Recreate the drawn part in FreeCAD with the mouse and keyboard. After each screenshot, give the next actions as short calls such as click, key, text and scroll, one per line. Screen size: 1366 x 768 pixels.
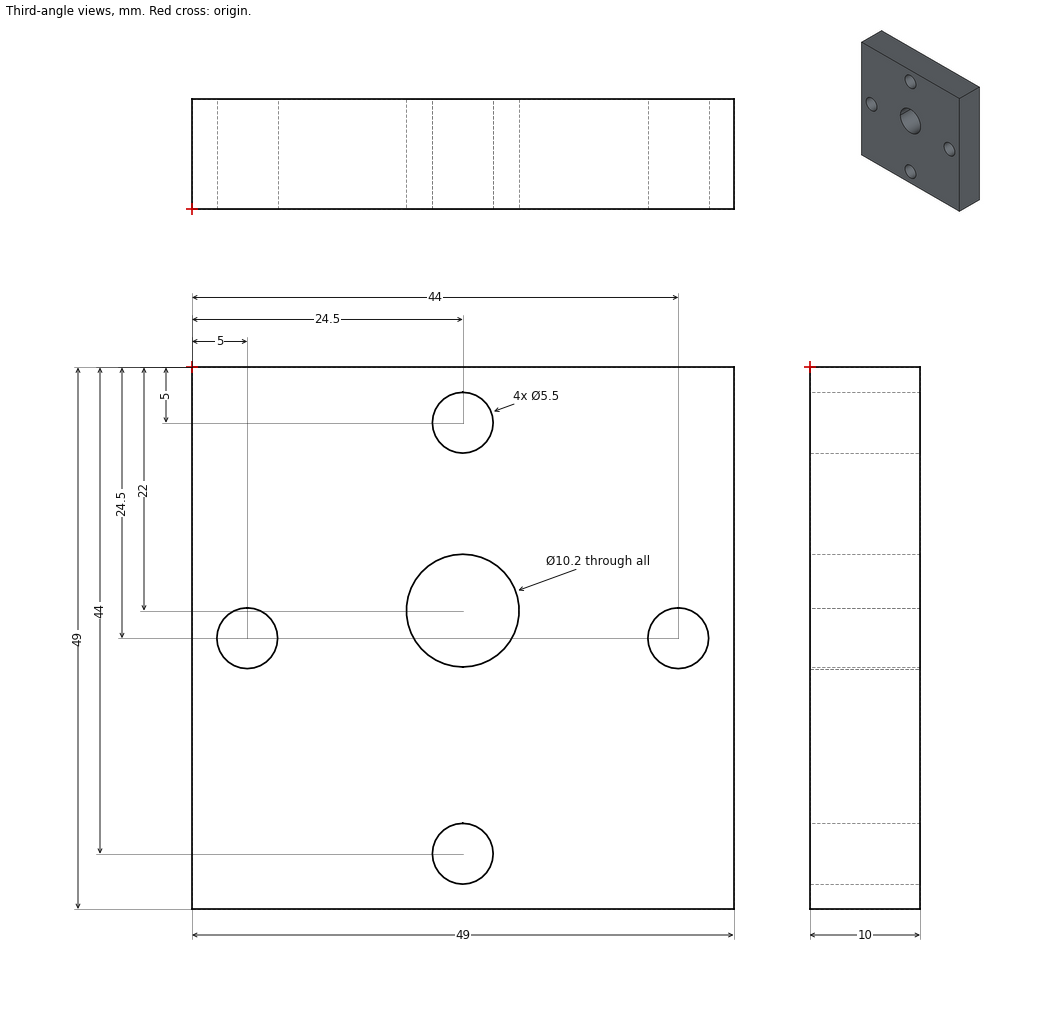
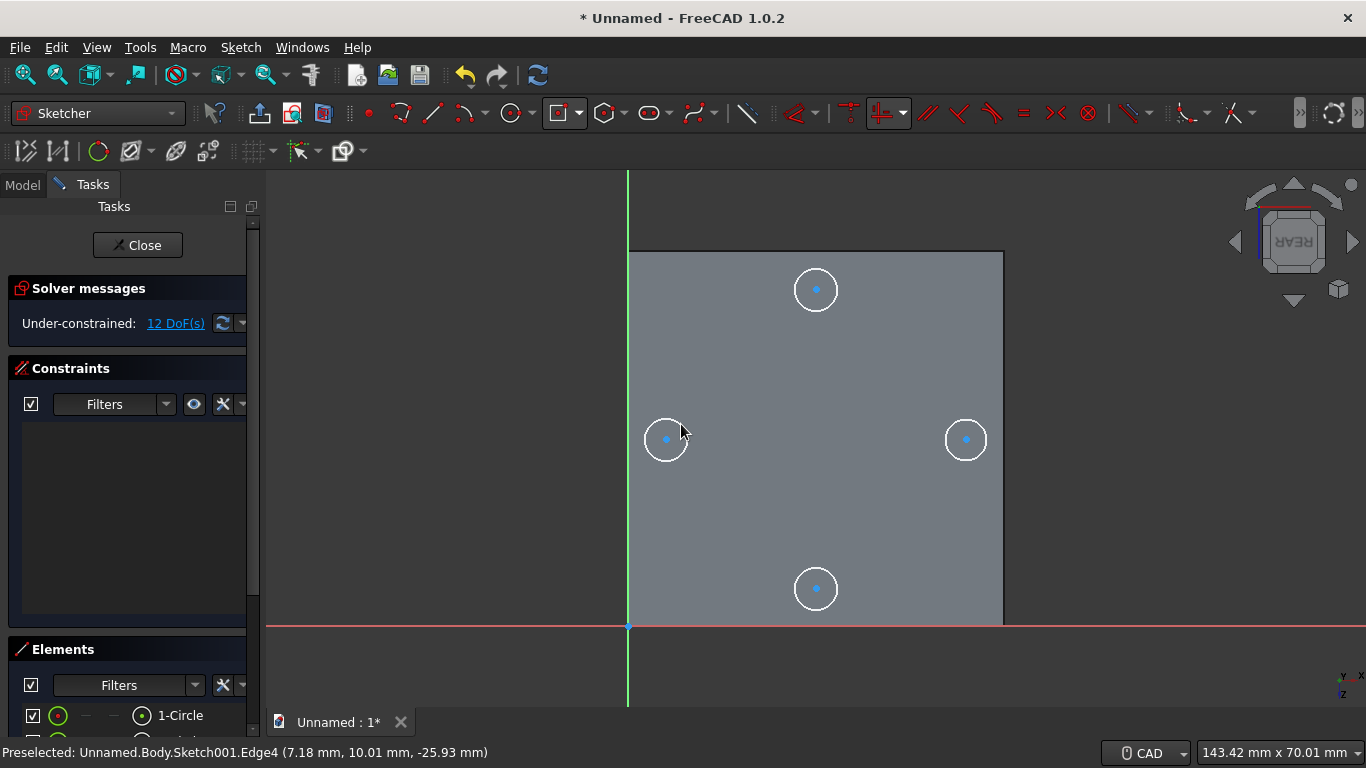
click(831, 574)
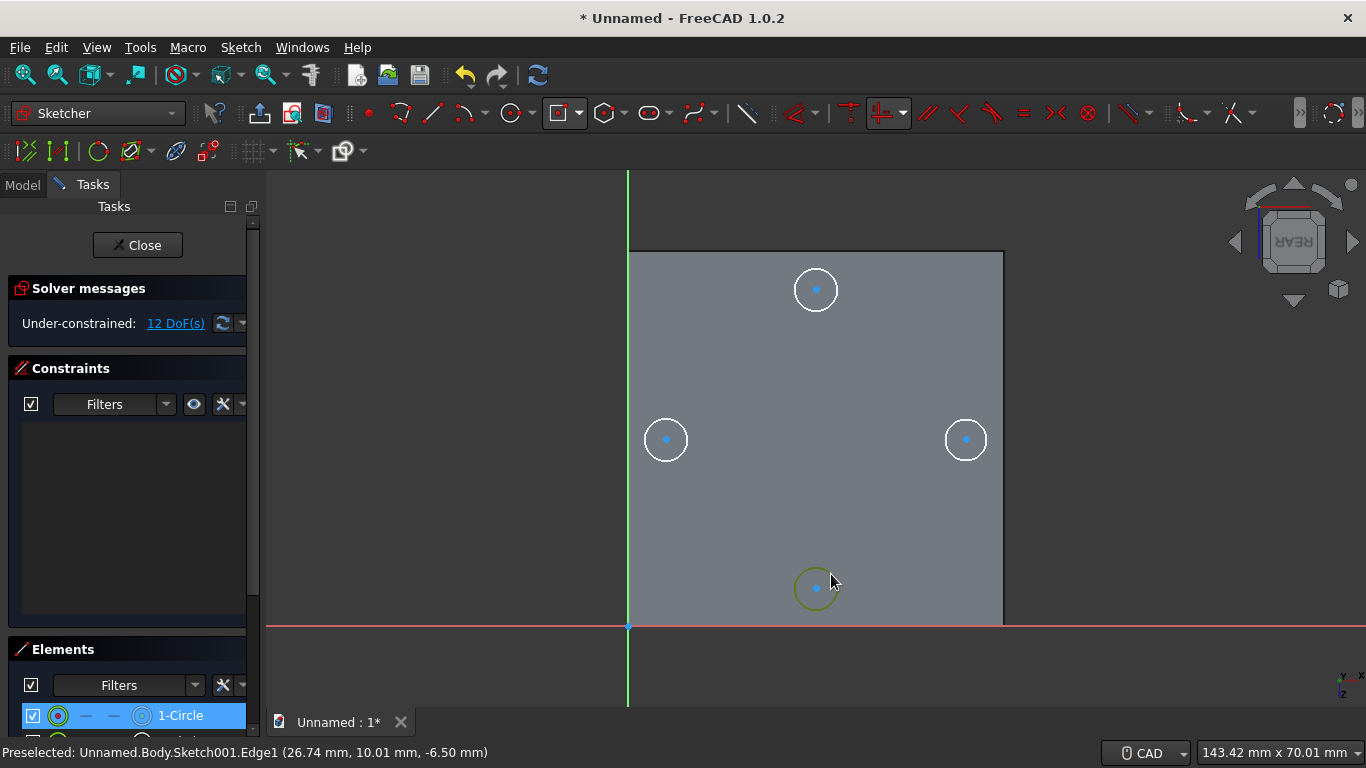
click(980, 425)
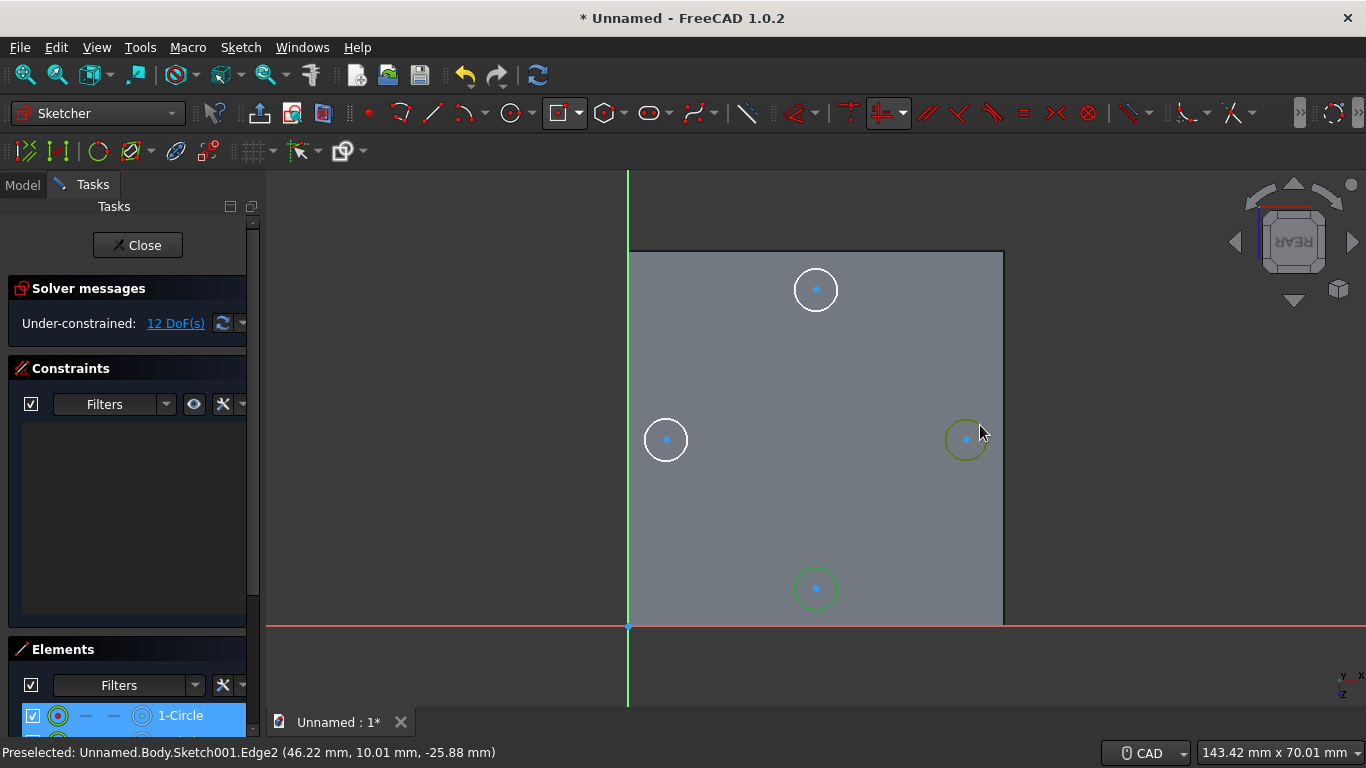
click(831, 275)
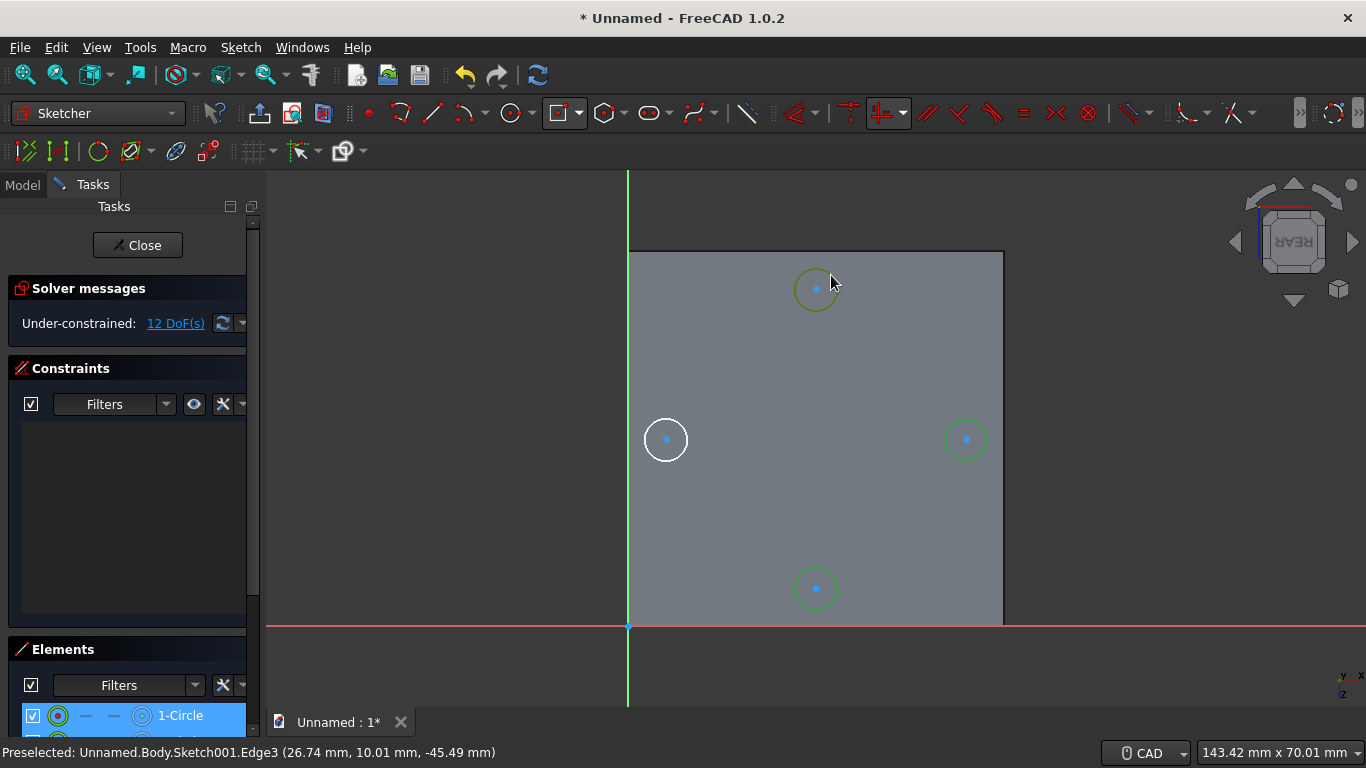
click(681, 425)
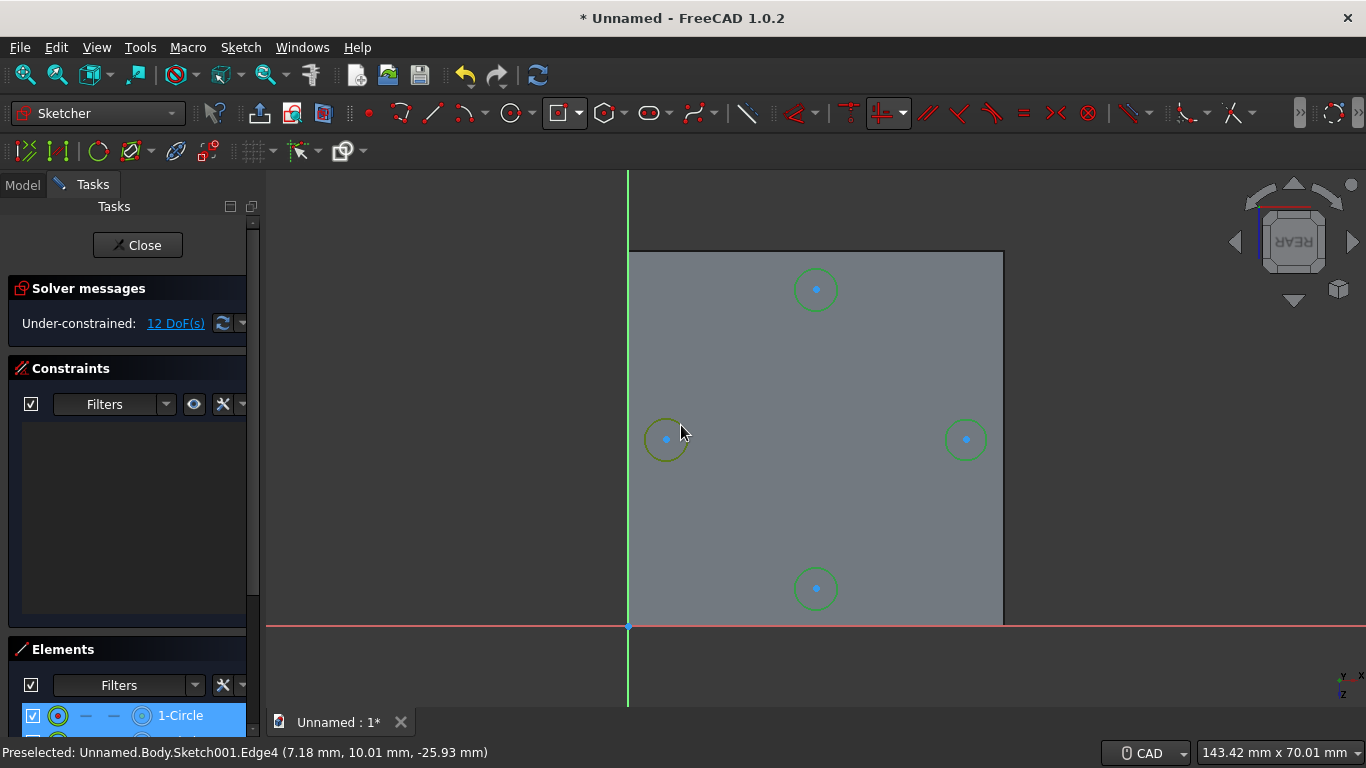
click(1024, 114)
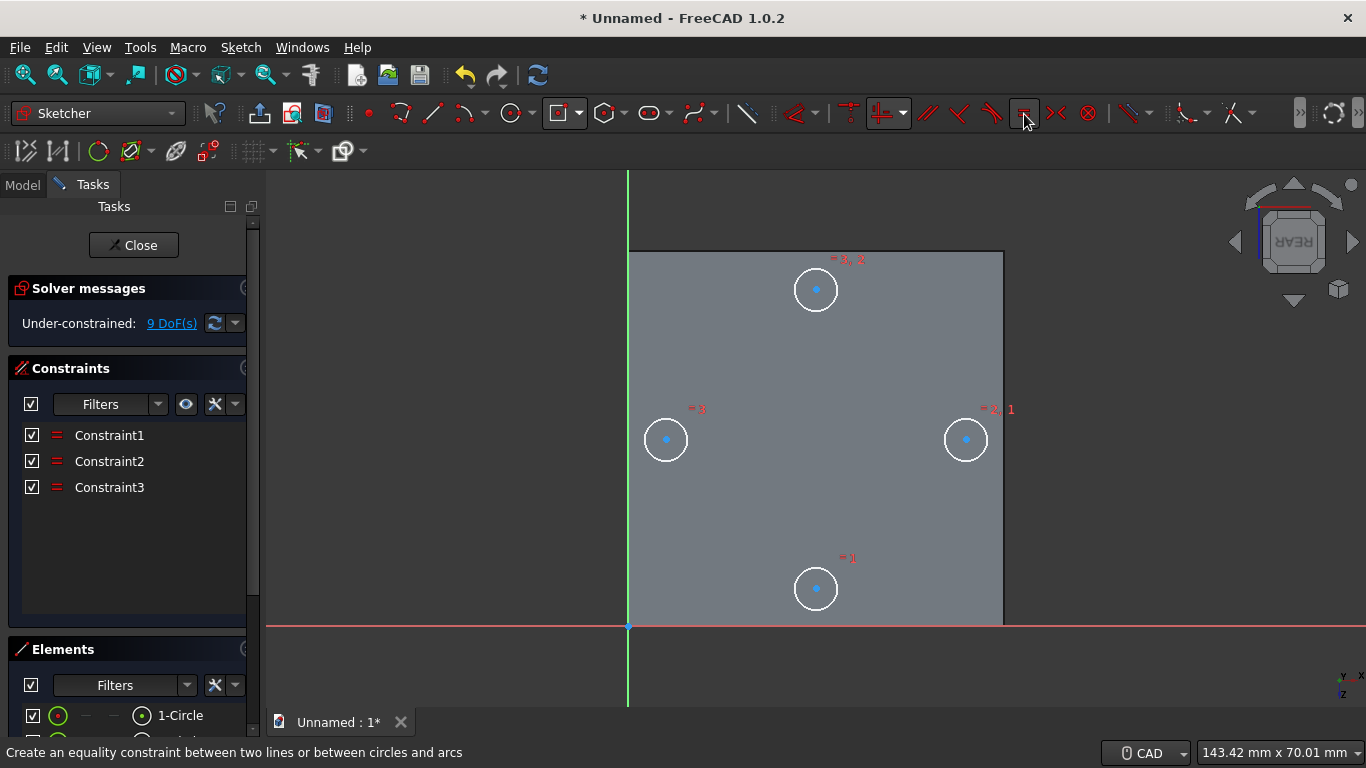
click(816, 589)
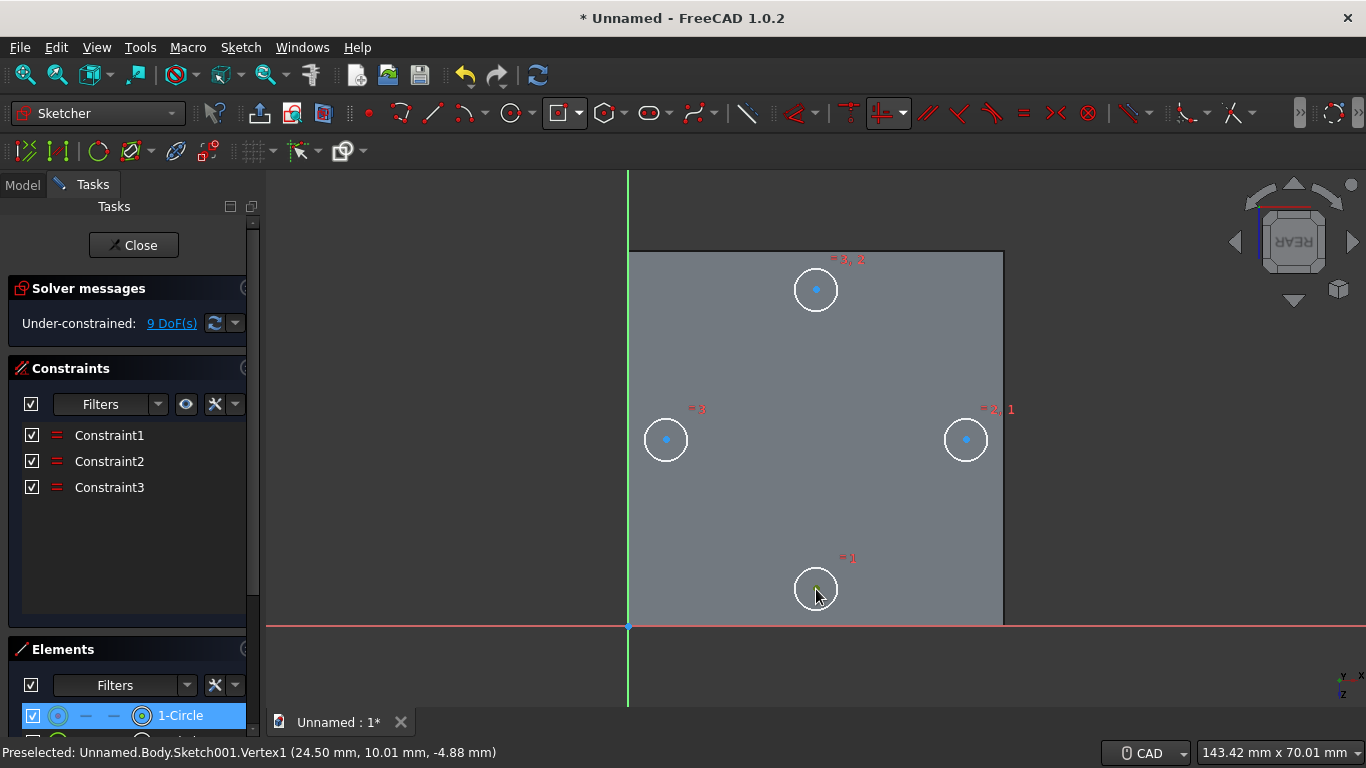
click(816, 290)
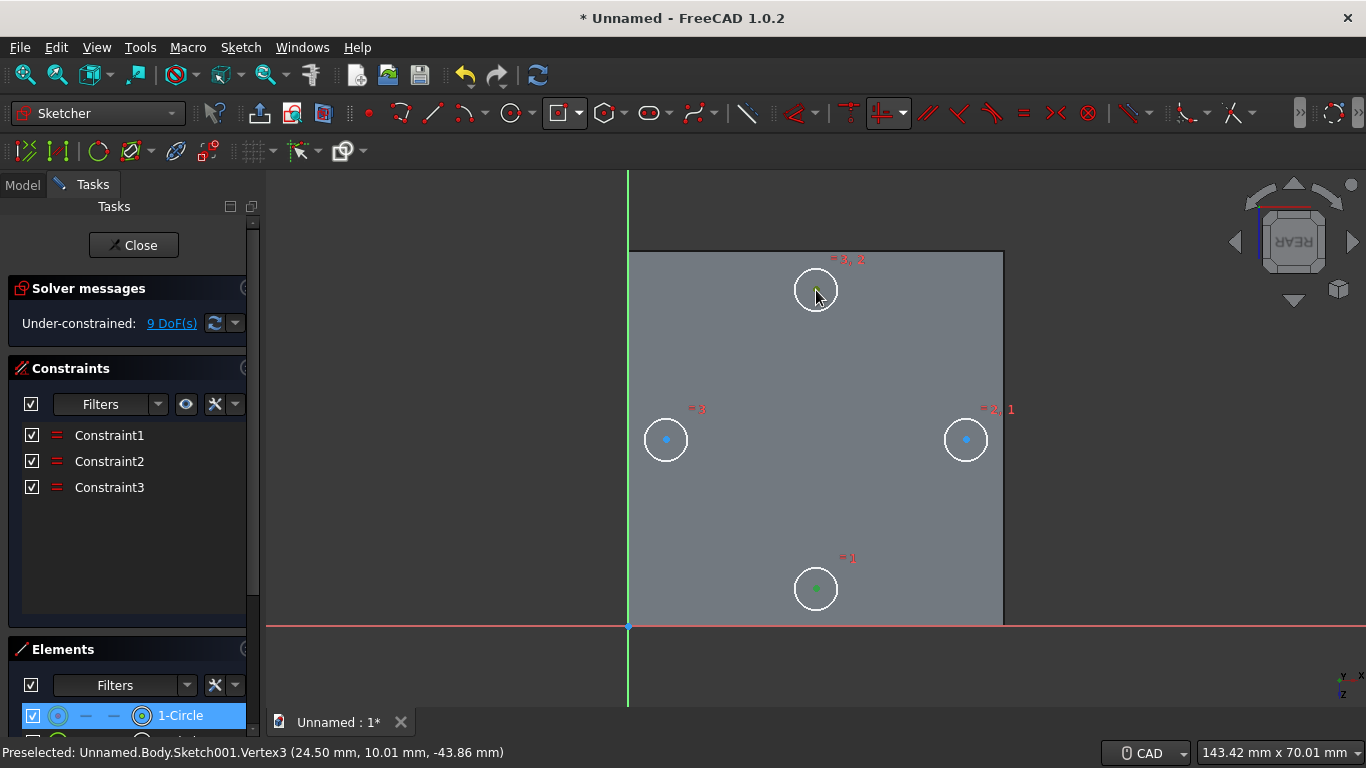
click(906, 114)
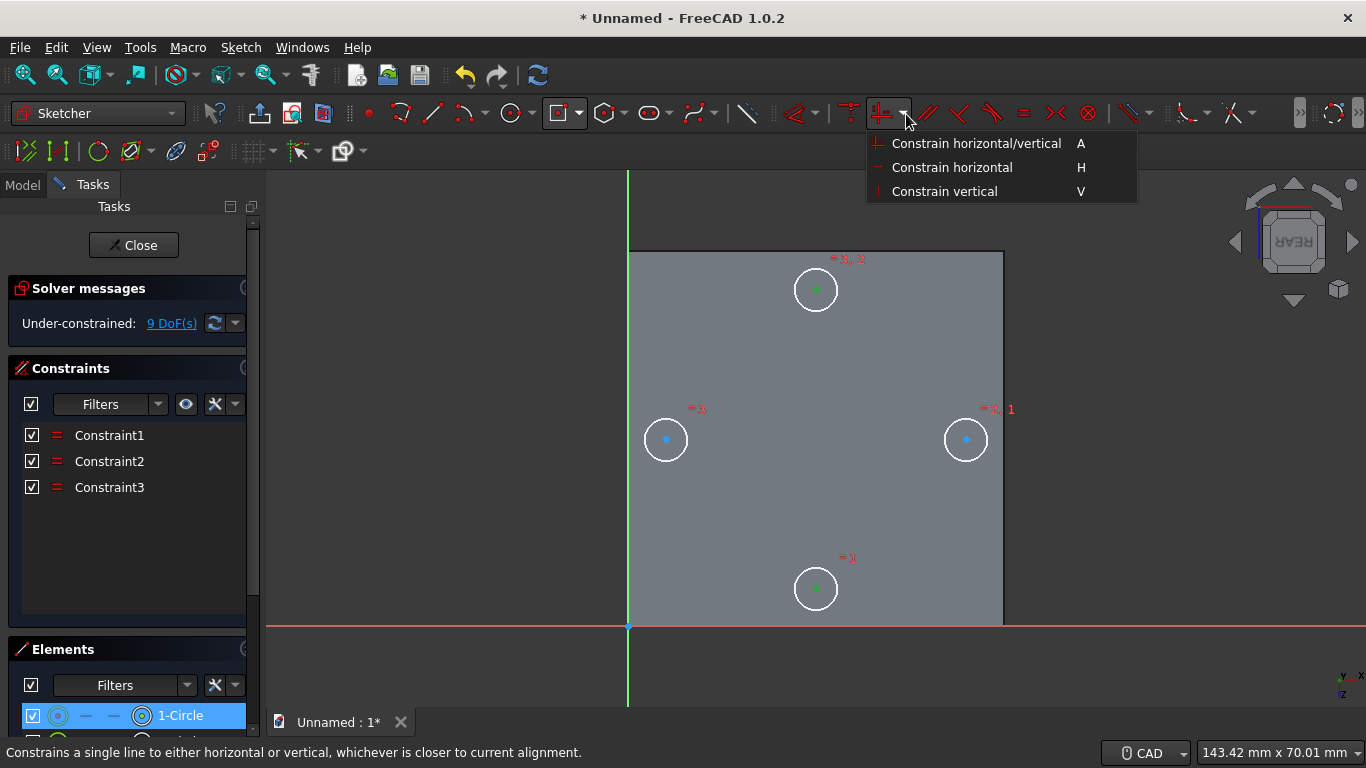
click(1002, 191)